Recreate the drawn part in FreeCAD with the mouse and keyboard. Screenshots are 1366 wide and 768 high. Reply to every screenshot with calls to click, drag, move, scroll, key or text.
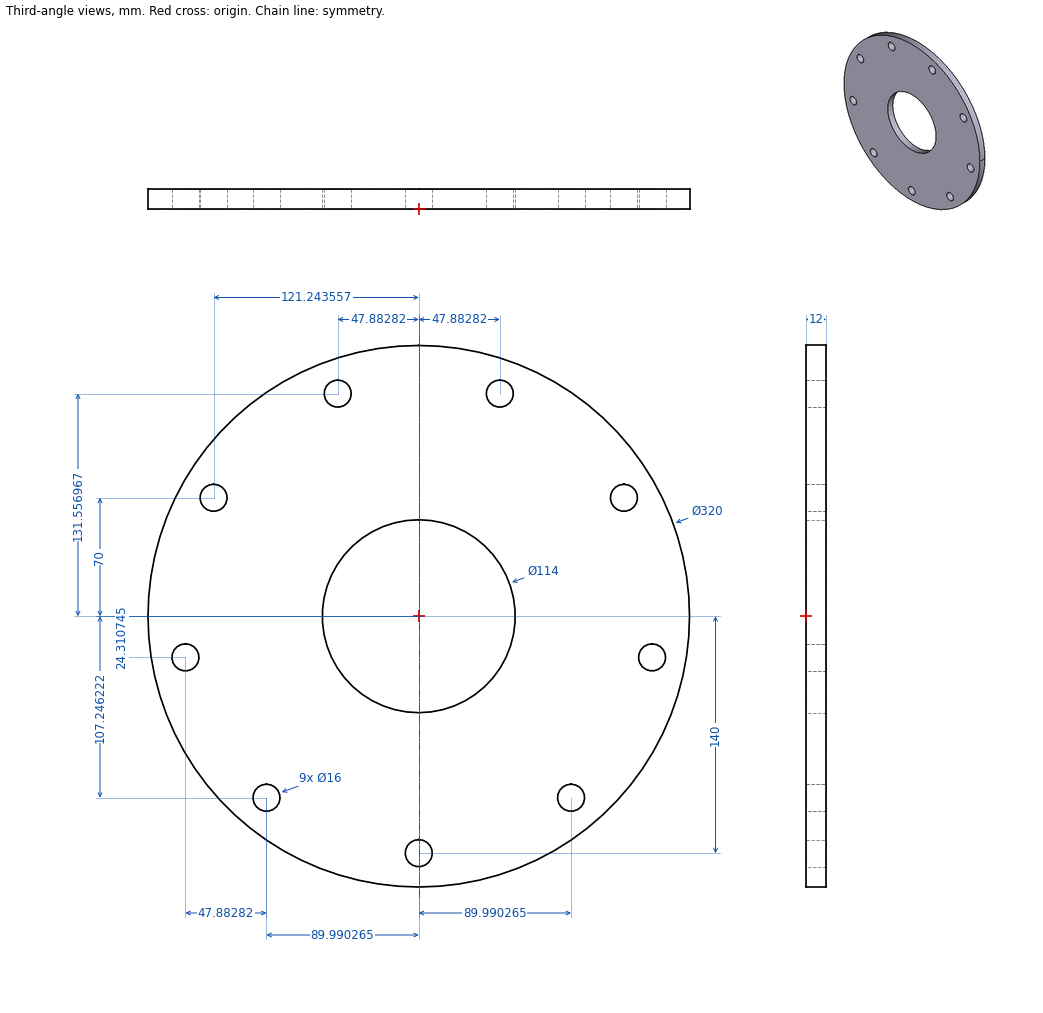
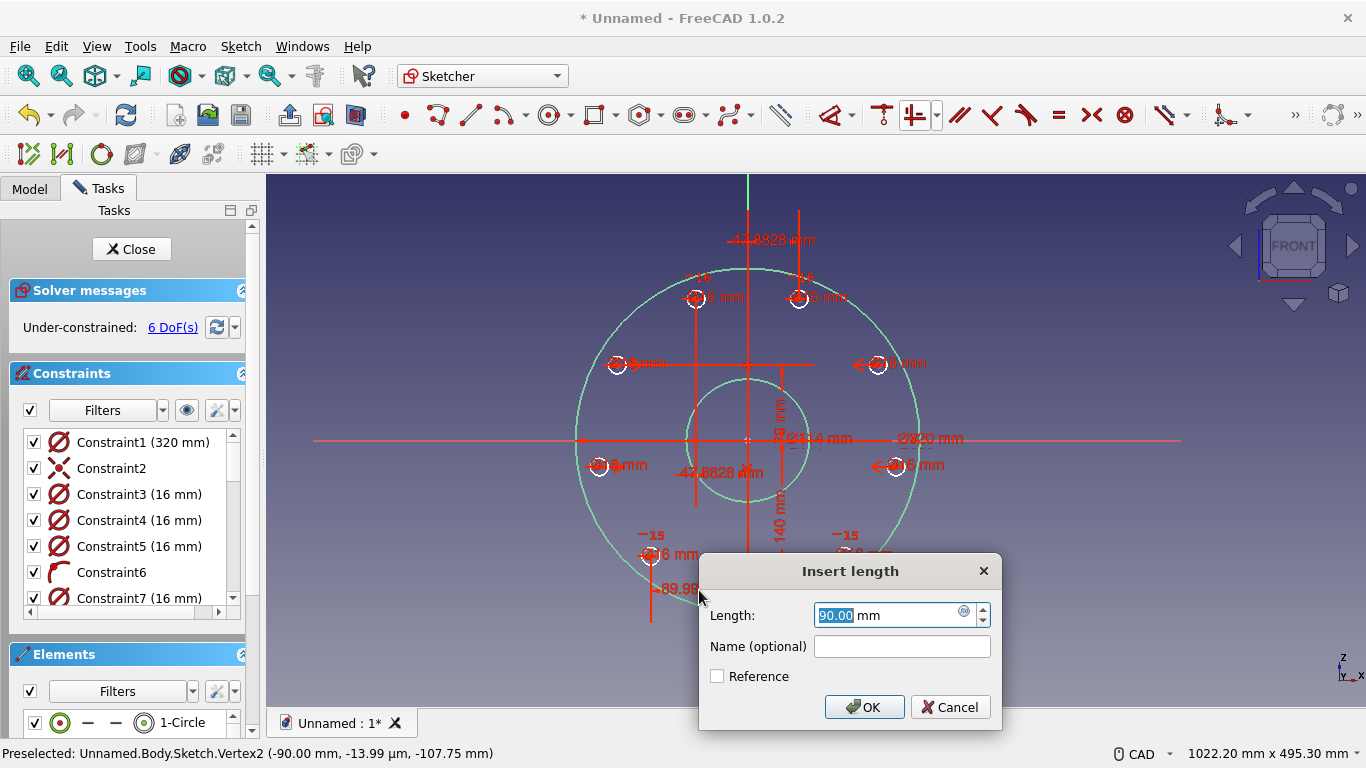
text(89.990265)
key(Return)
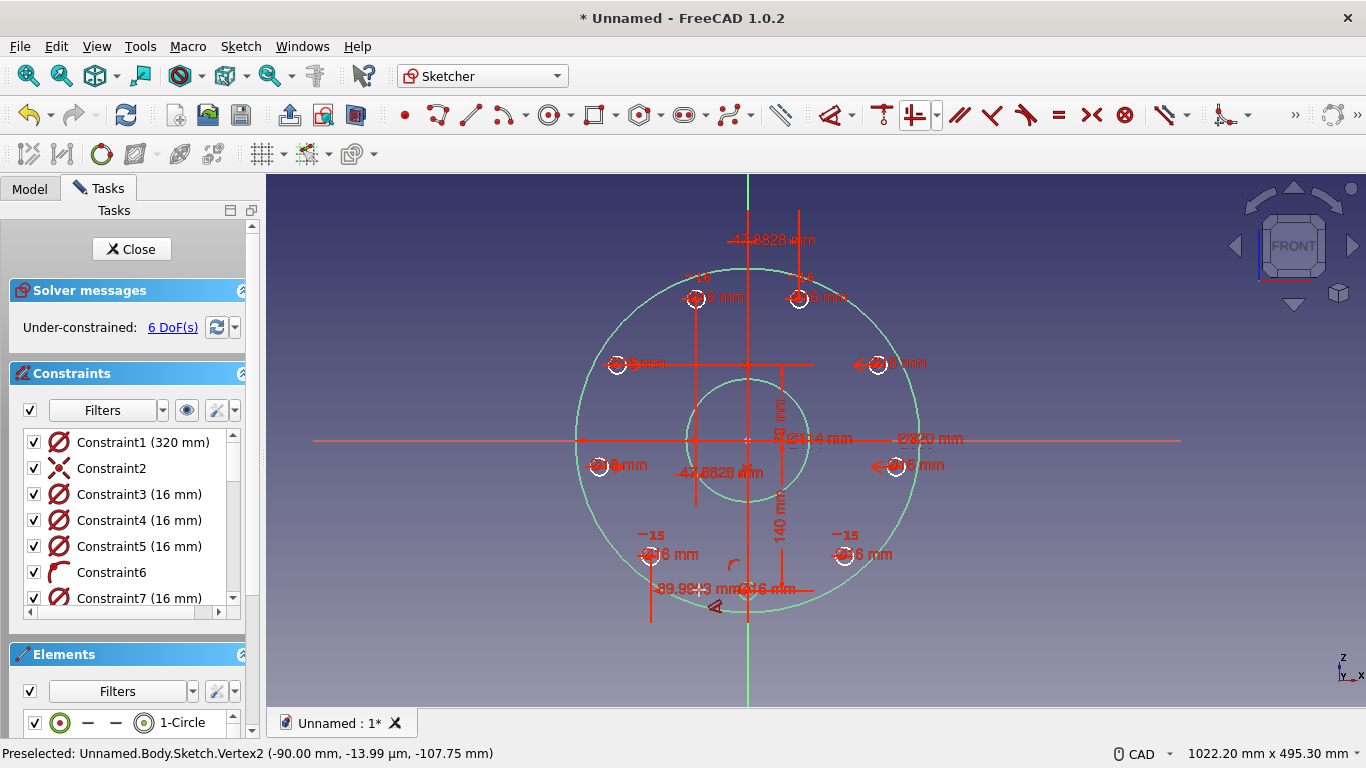
scroll(599, 467, up, 3)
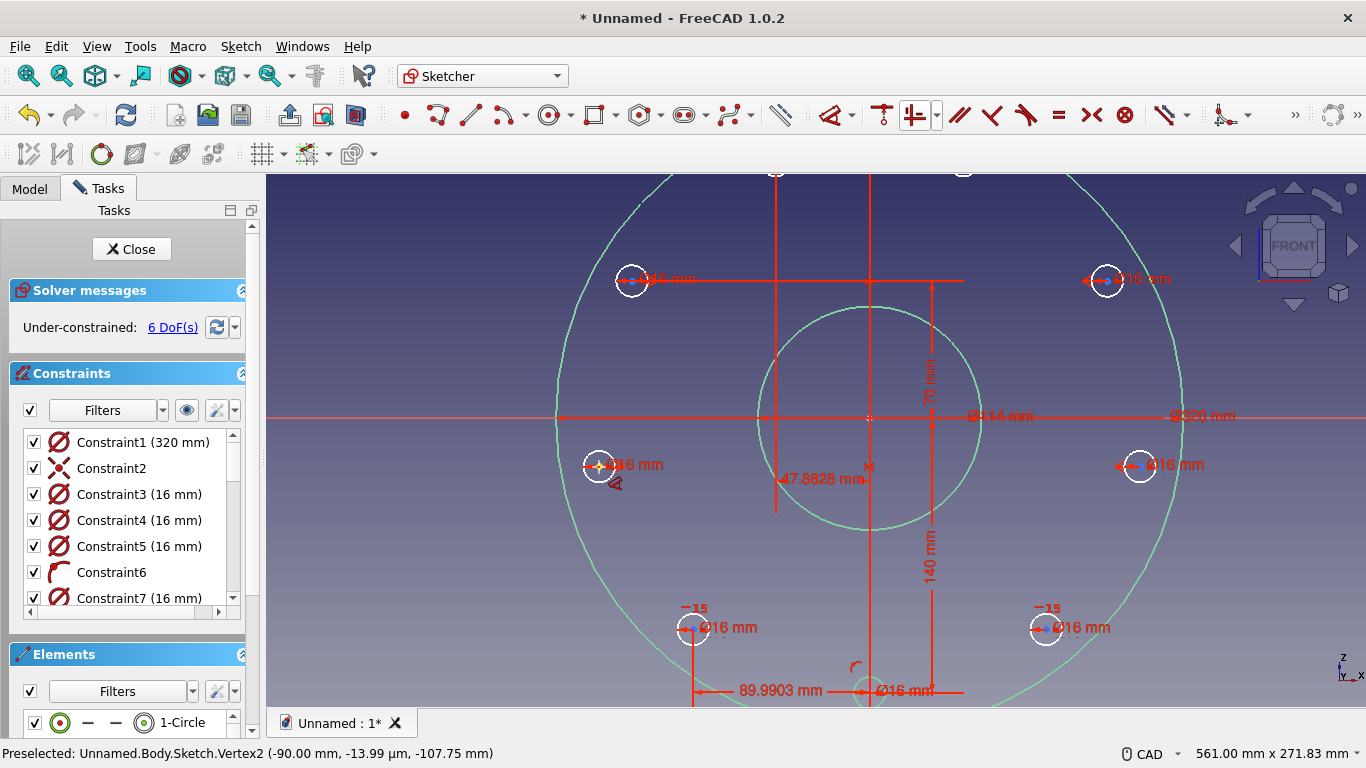
click(599, 467)
click(904, 442)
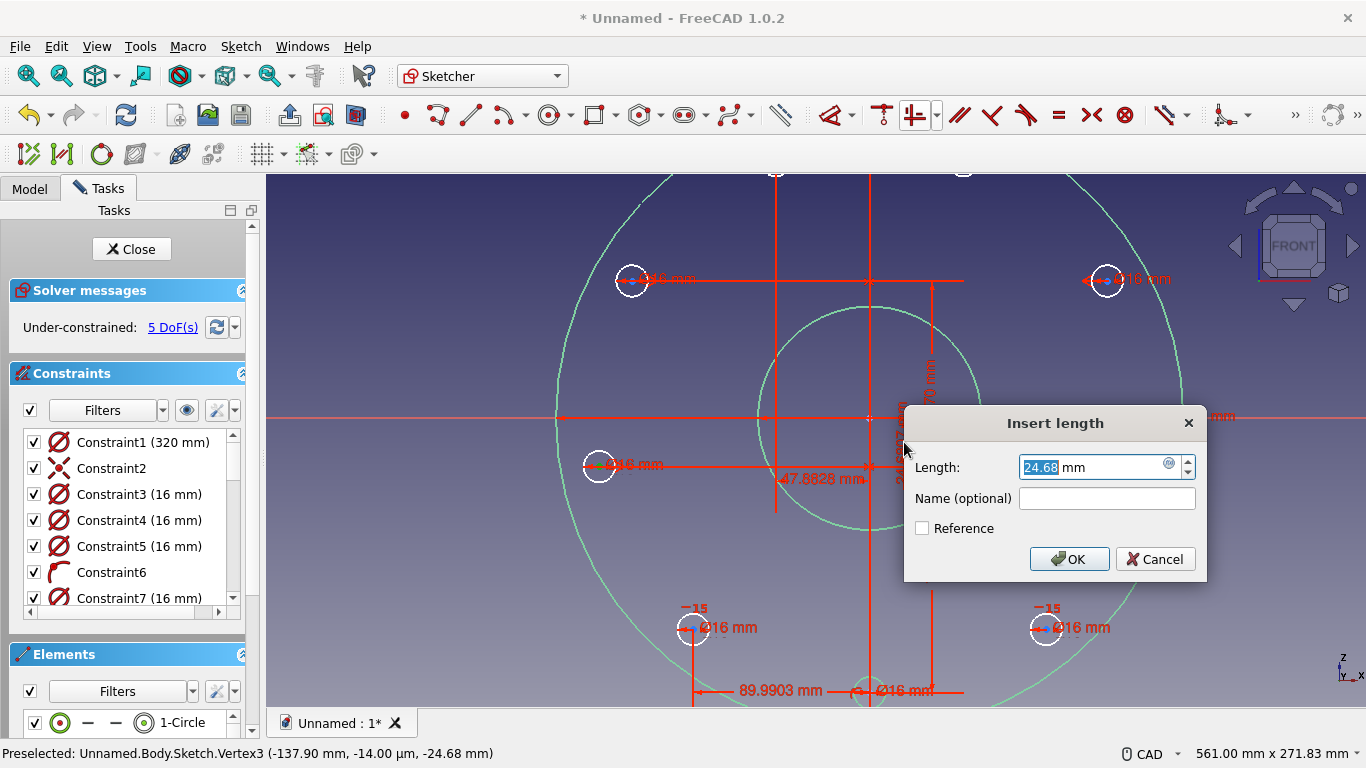
text(24.310745)
key(Return)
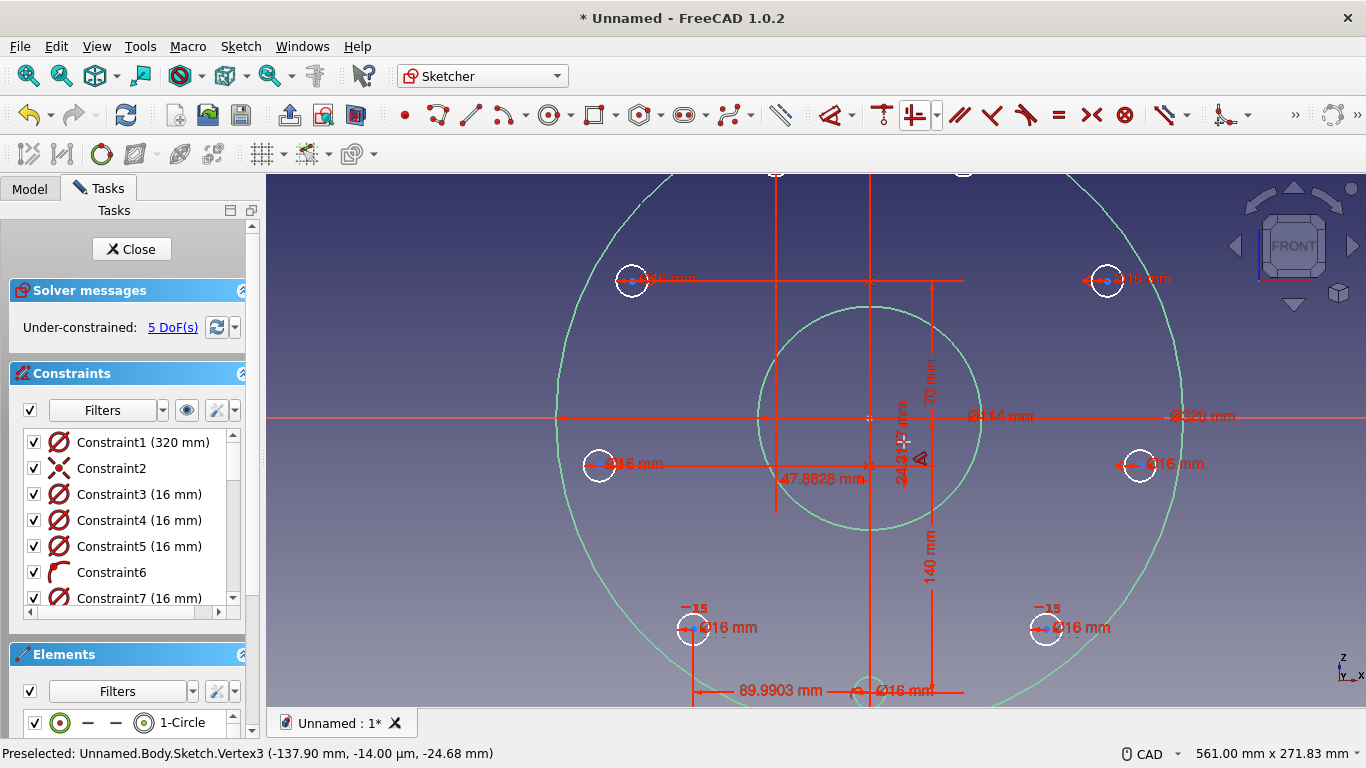
click(1046, 630)
click(958, 664)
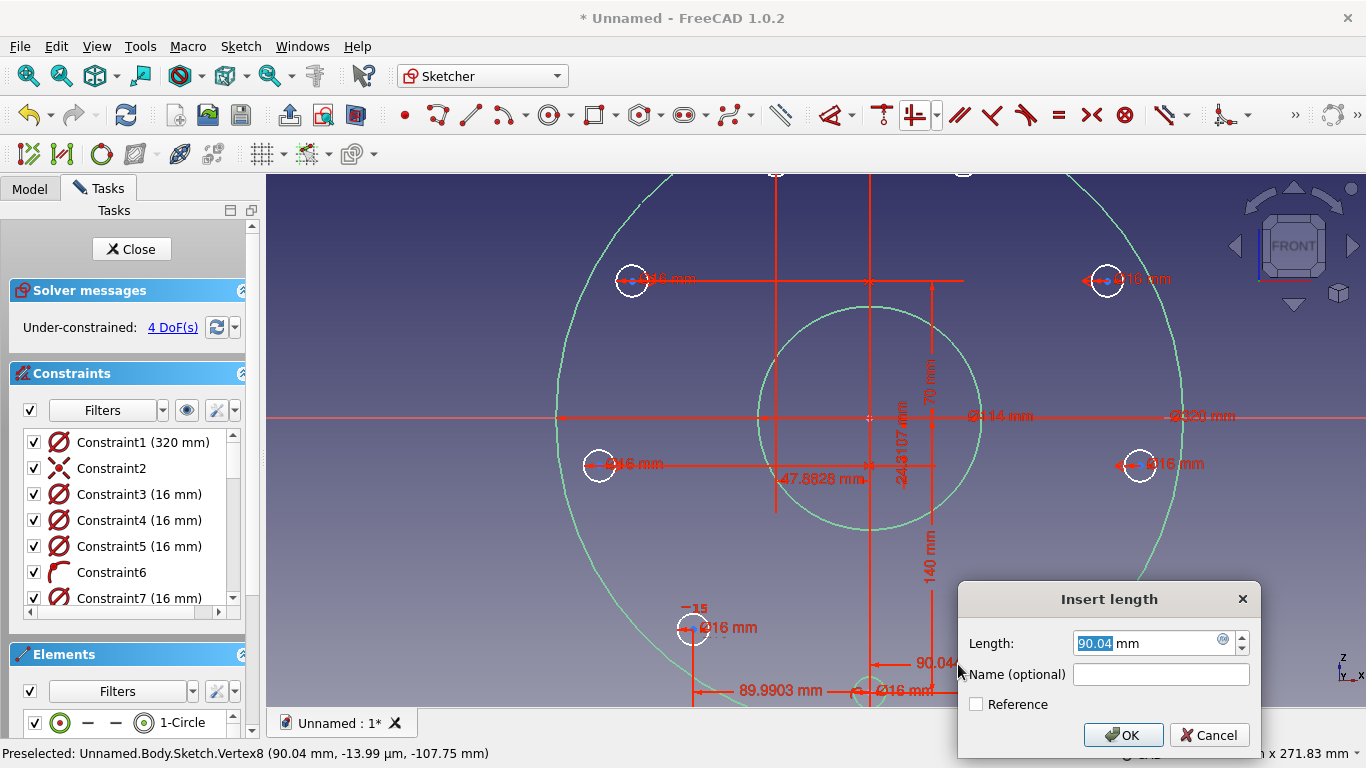
text(89.990265)
key(Return)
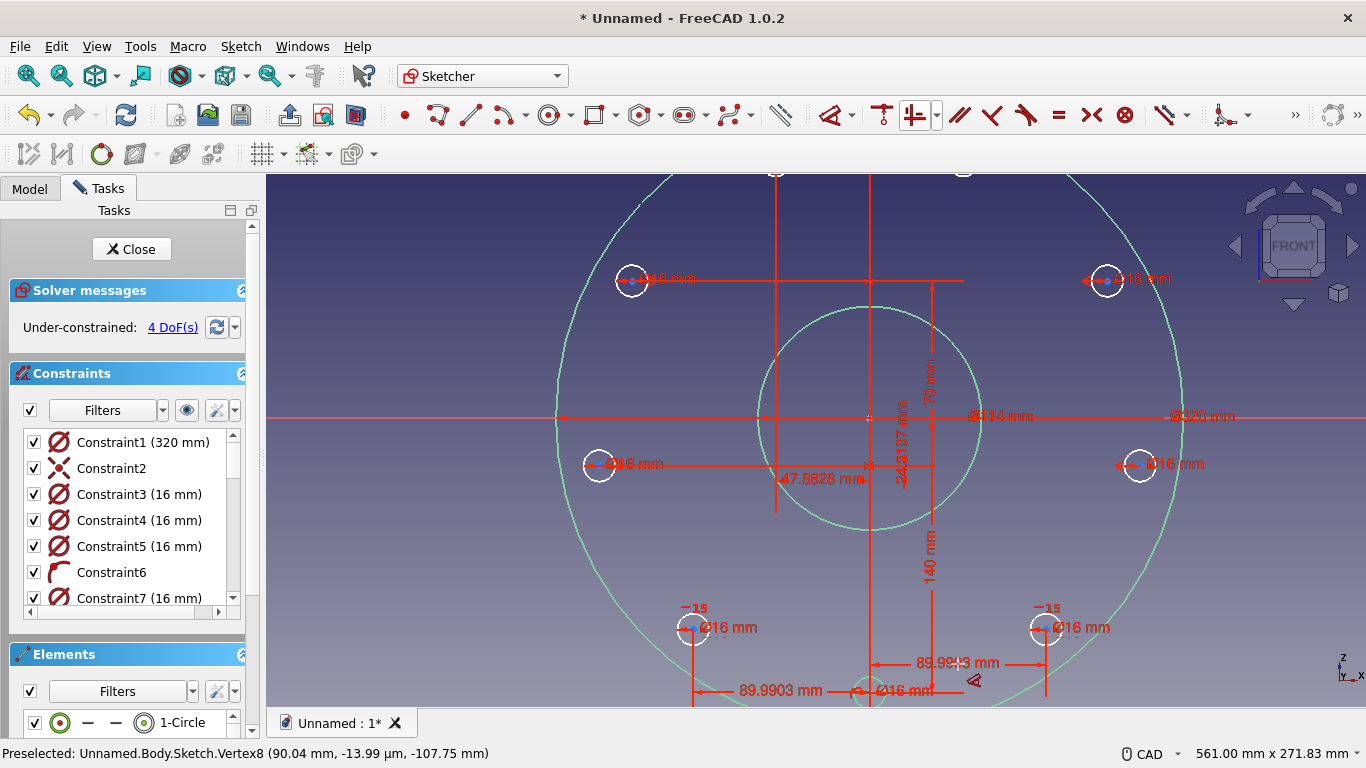
click(693, 630)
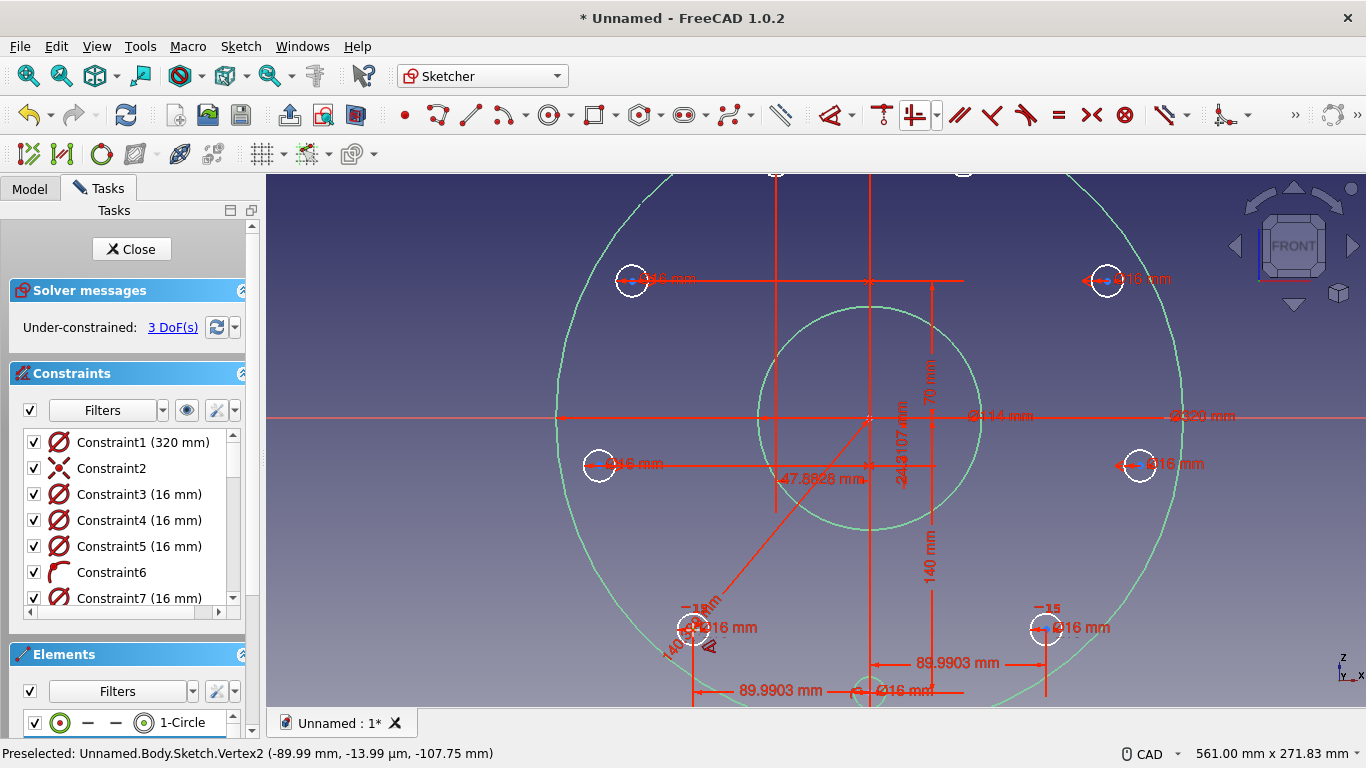
click(599, 466)
click(646, 664)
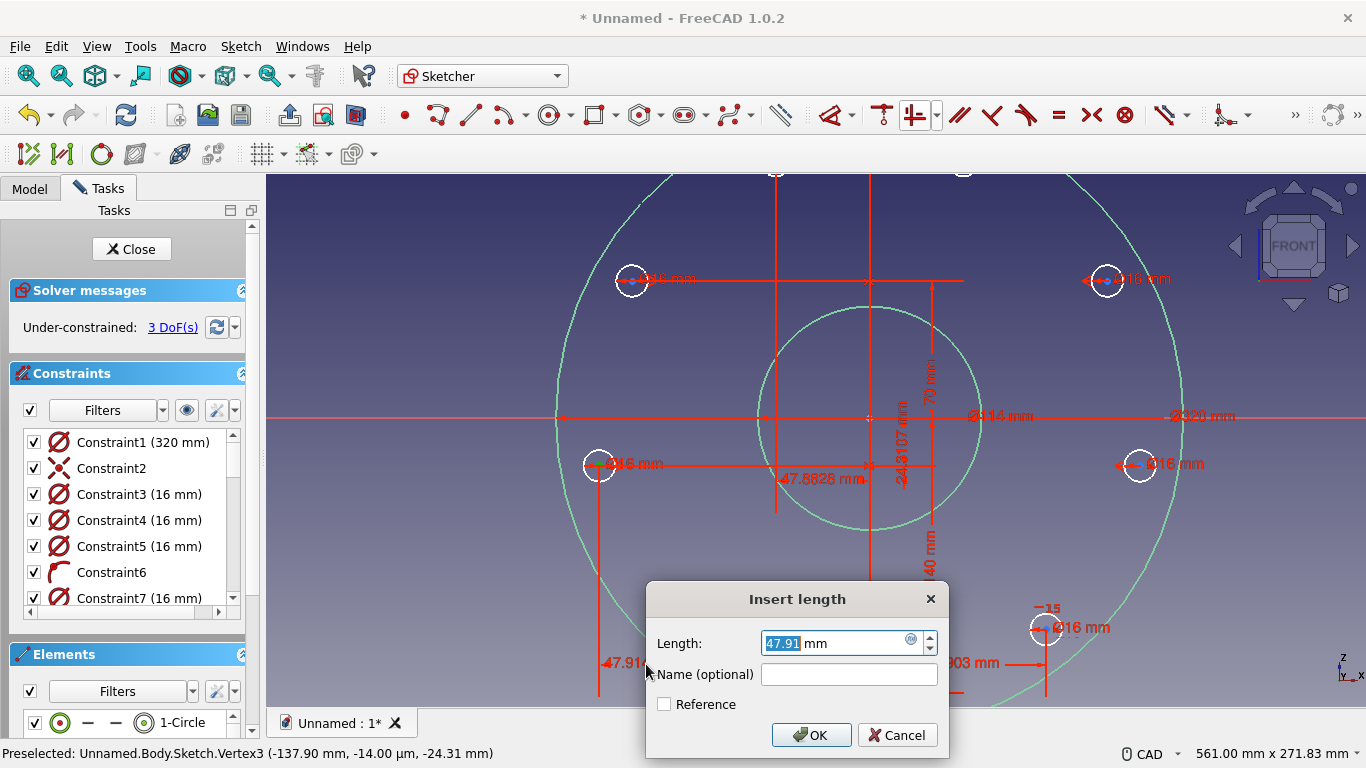
text(47.88282)
key(Return)